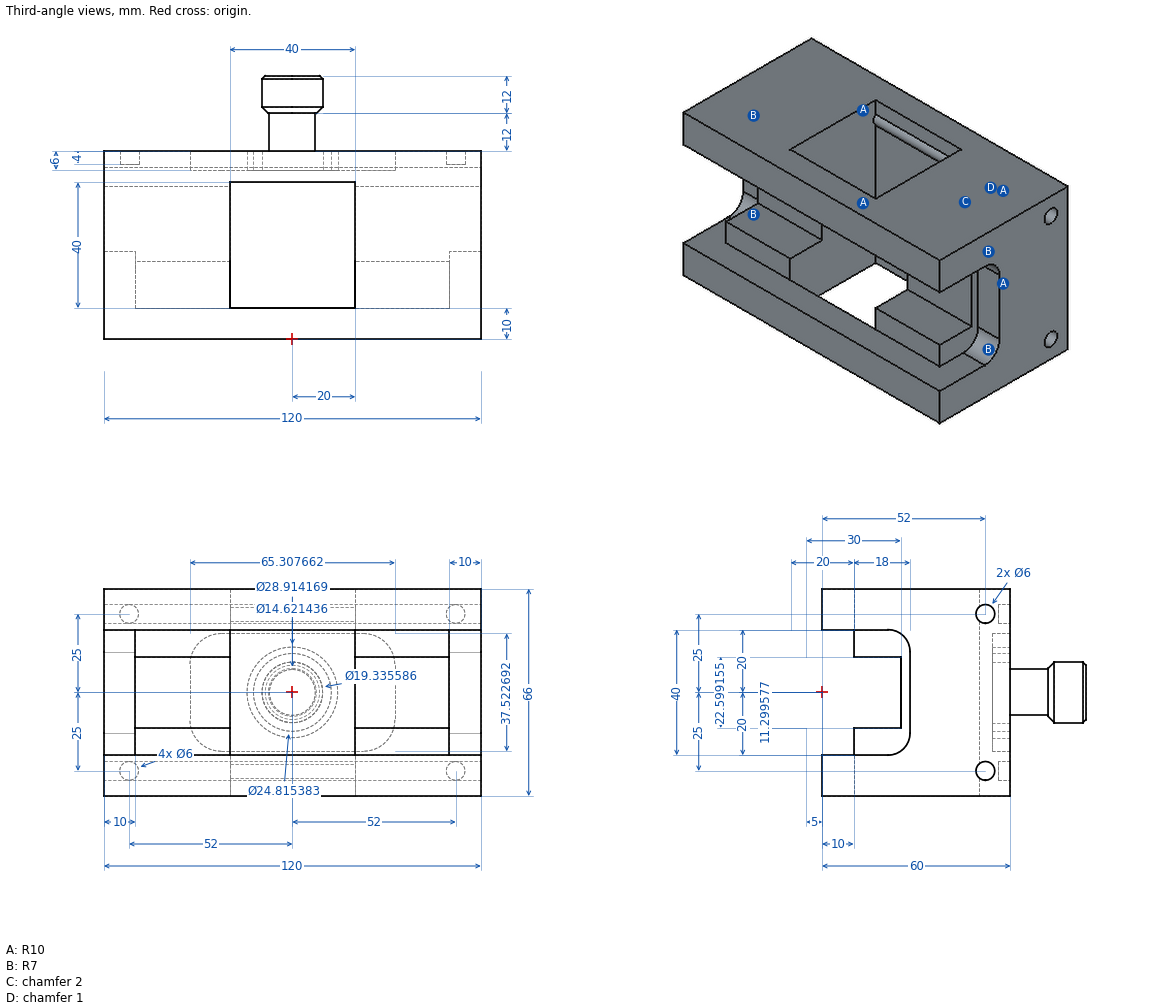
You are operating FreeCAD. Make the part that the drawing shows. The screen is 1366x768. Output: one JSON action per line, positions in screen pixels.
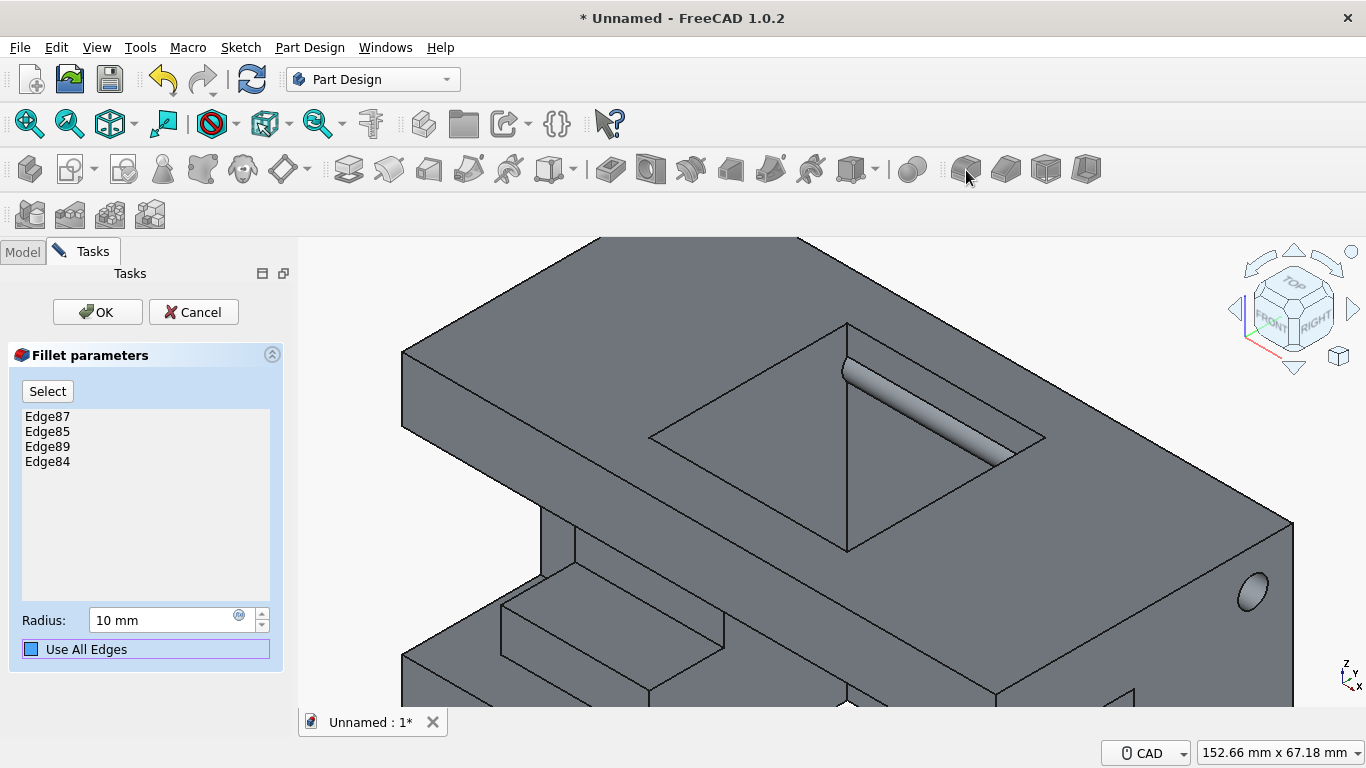
{"action": "left_click", "coordinate": [98, 312]}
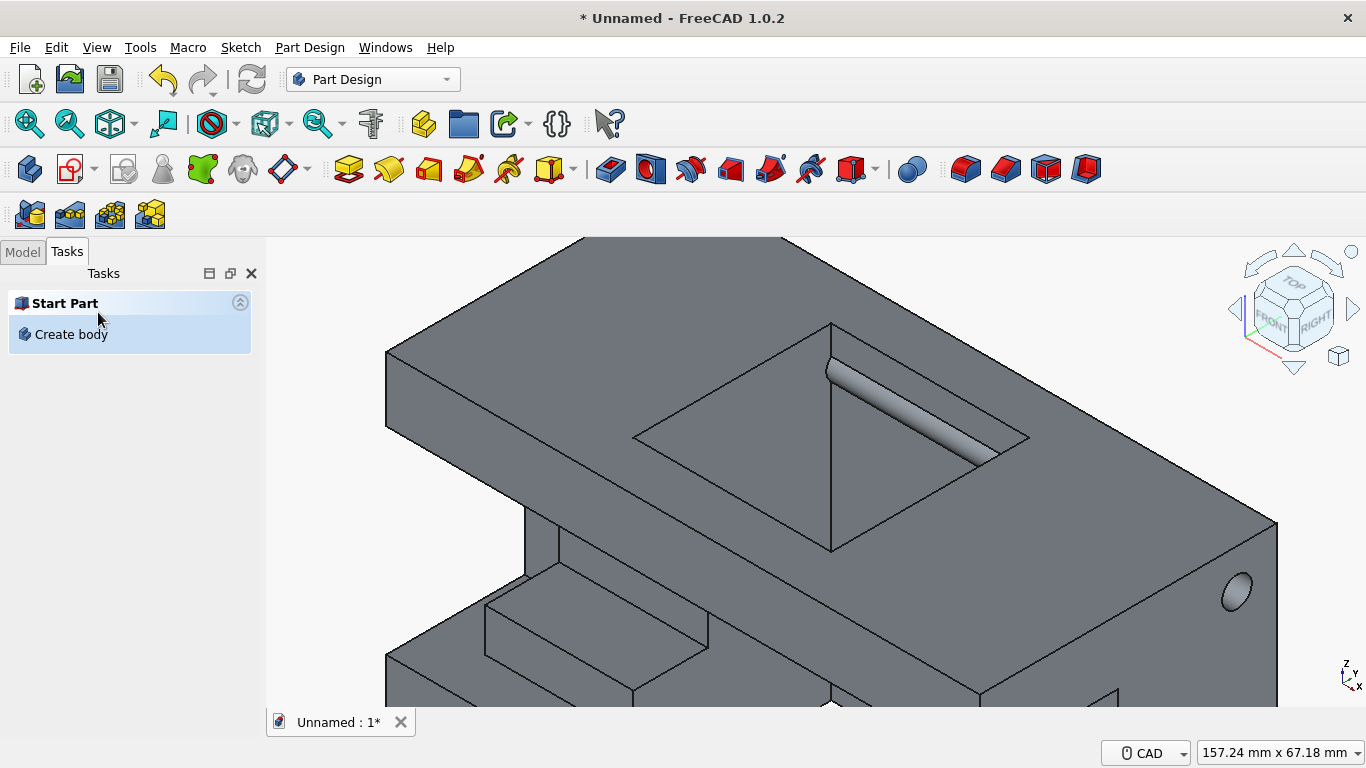
{"action": "left_click", "coordinate": [30, 124]}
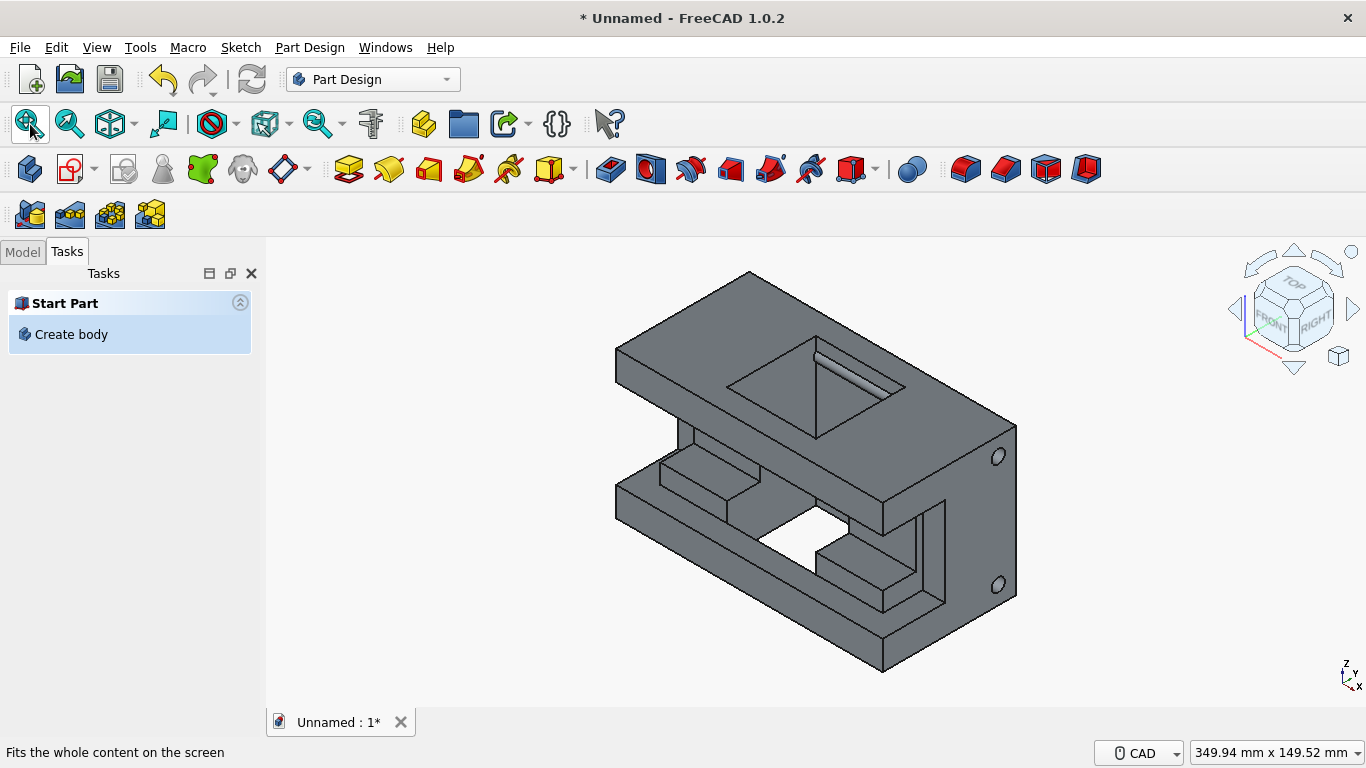
{"action": "key", "text": "4"}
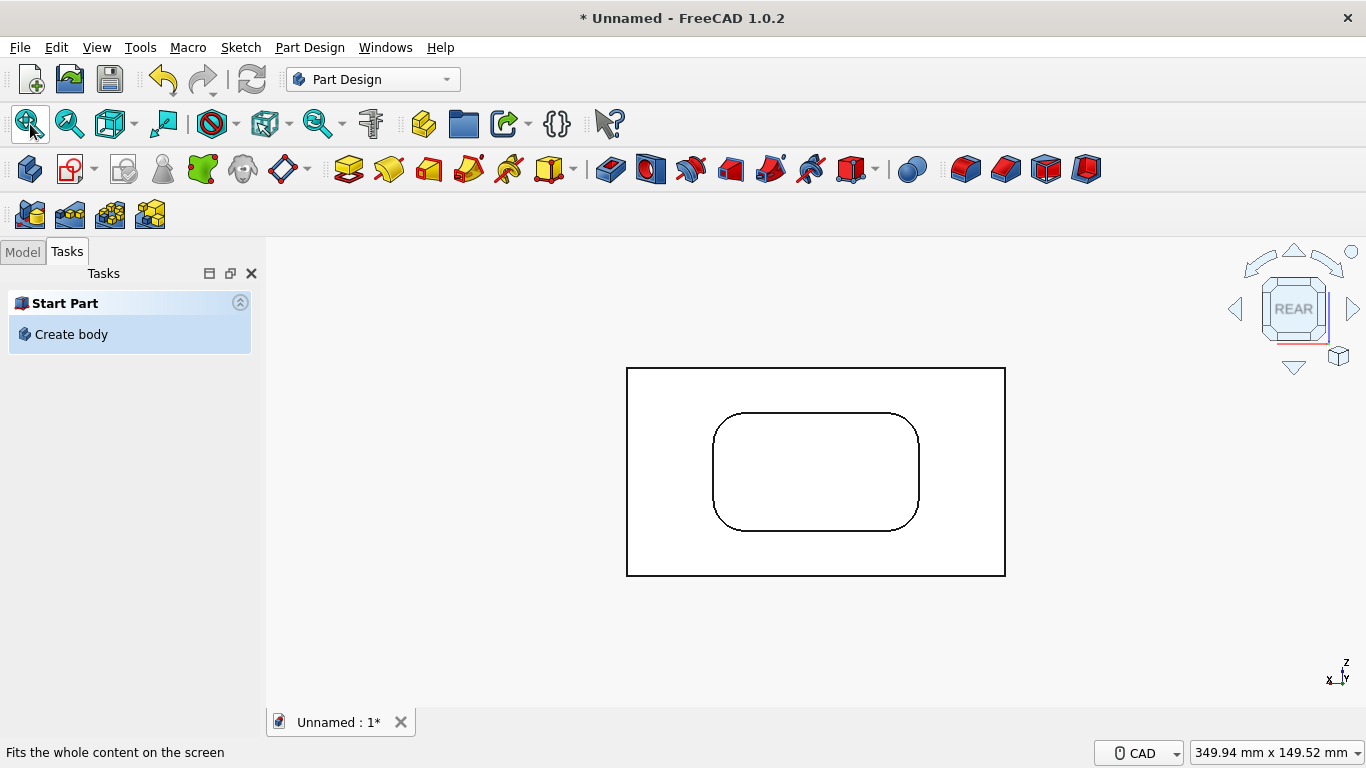
{"action": "left_click", "coordinate": [30, 124]}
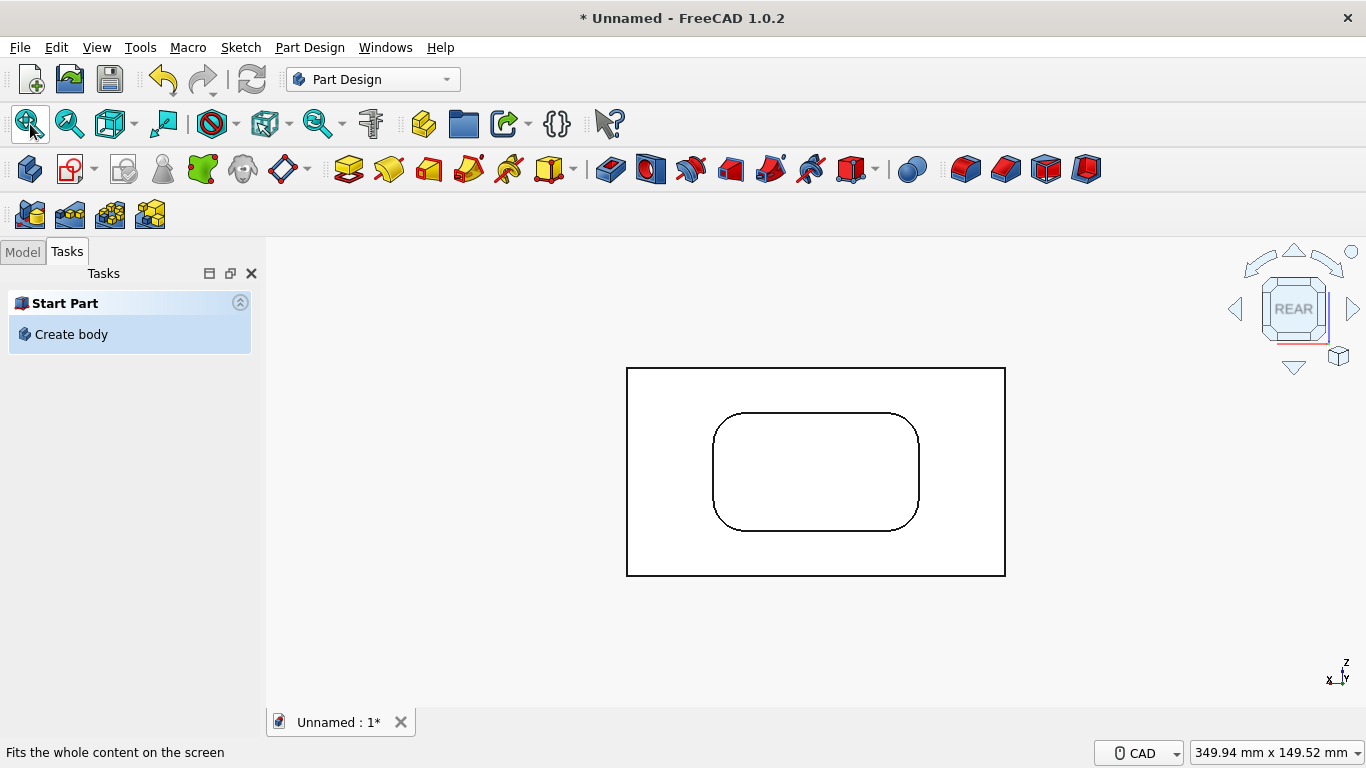
{"action": "left_click", "coordinate": [654, 412]}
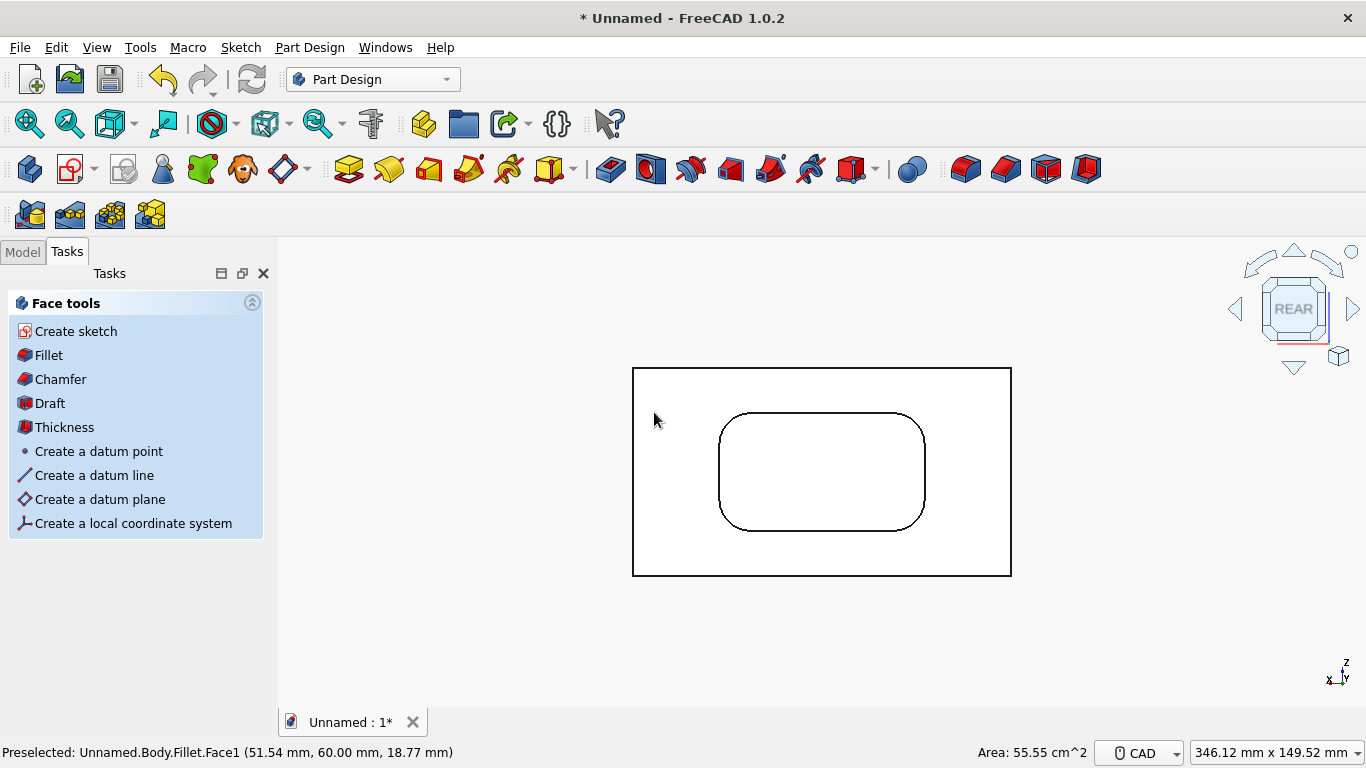
{"action": "left_click", "coordinate": [70, 170]}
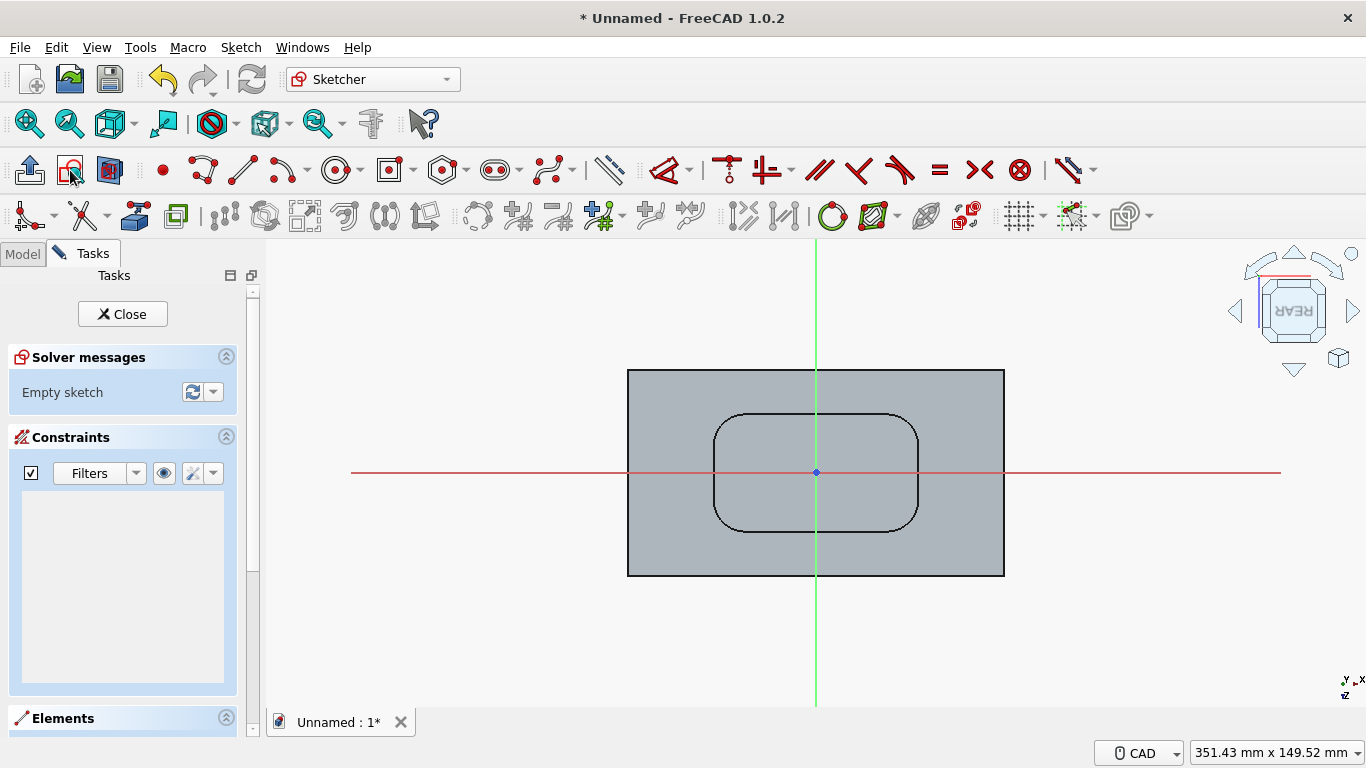
{"action": "scroll", "coordinate": [899, 473], "scroll_direction": "up", "scroll_amount": 3}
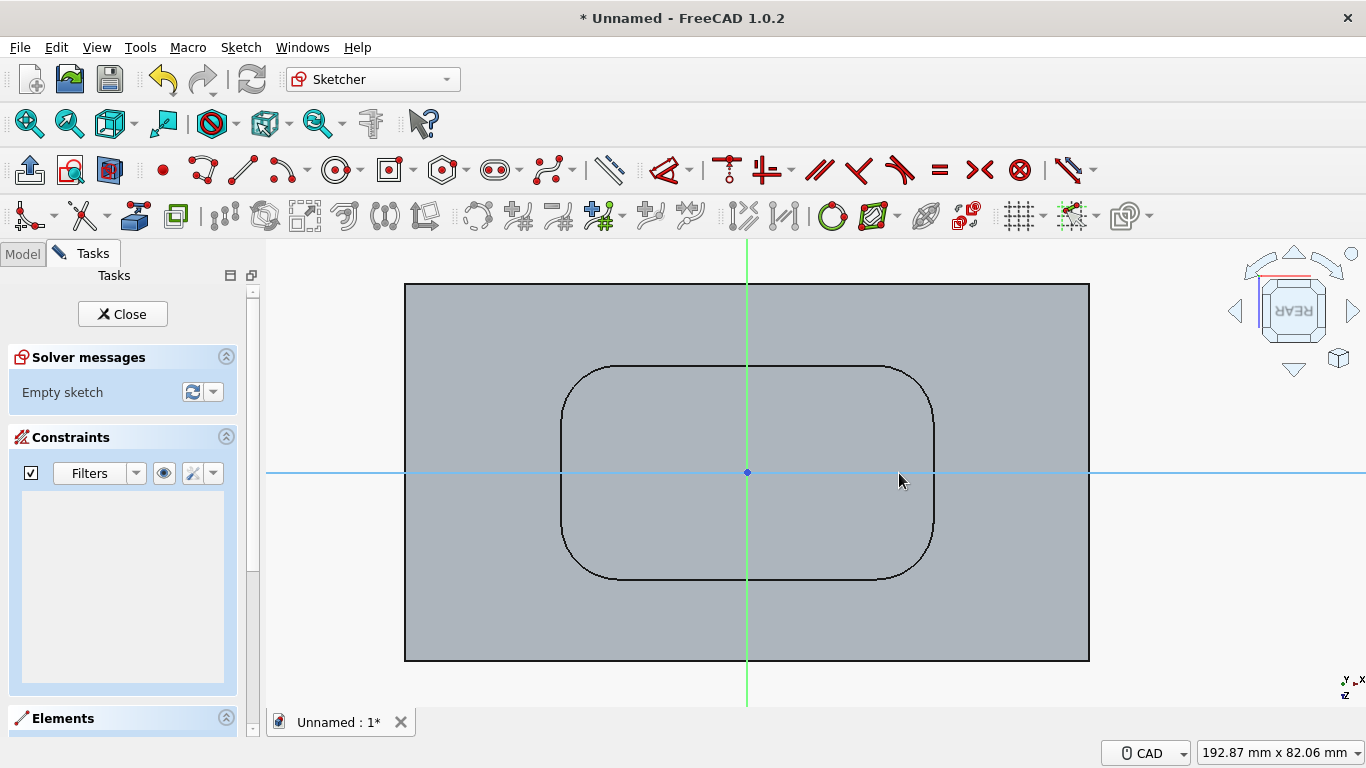
{"action": "left_click", "coordinate": [336, 170]}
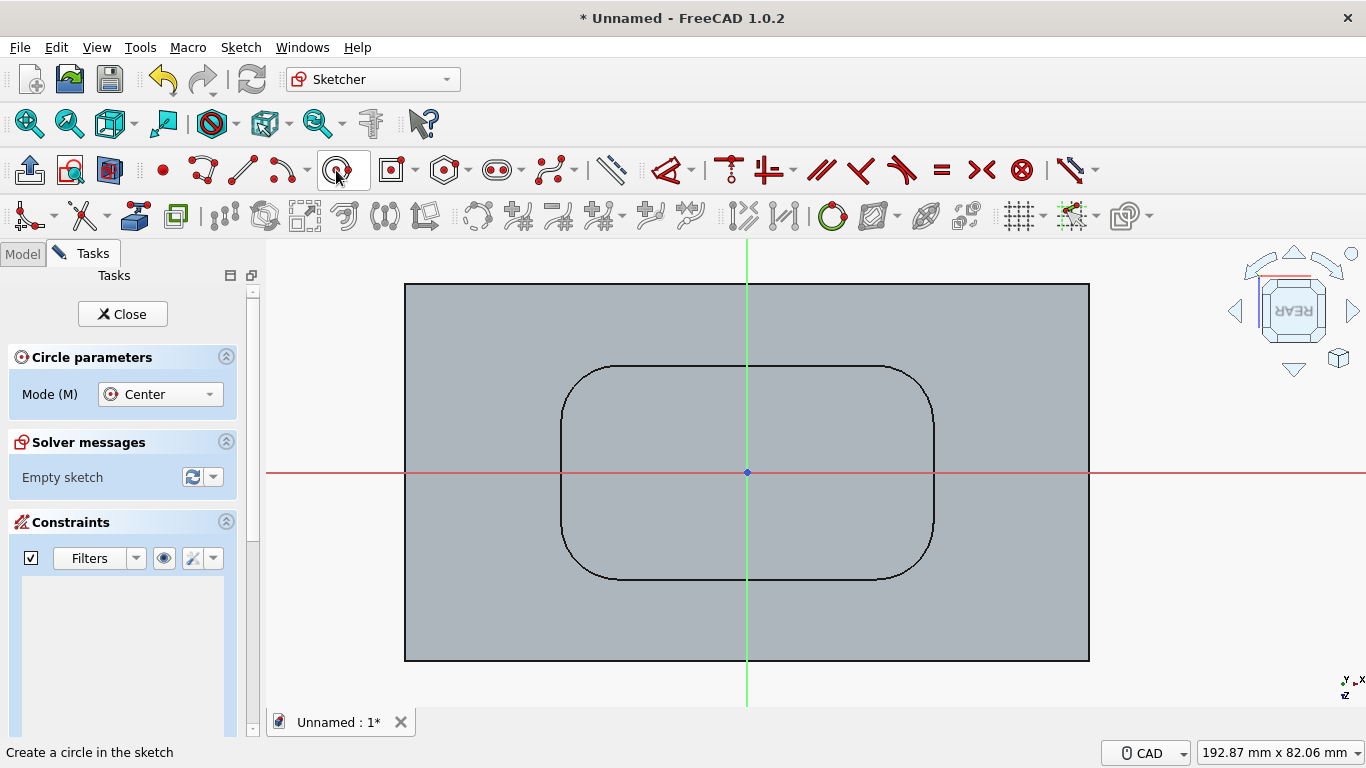
{"action": "scroll", "coordinate": [451, 330], "scroll_direction": "up", "scroll_amount": 2}